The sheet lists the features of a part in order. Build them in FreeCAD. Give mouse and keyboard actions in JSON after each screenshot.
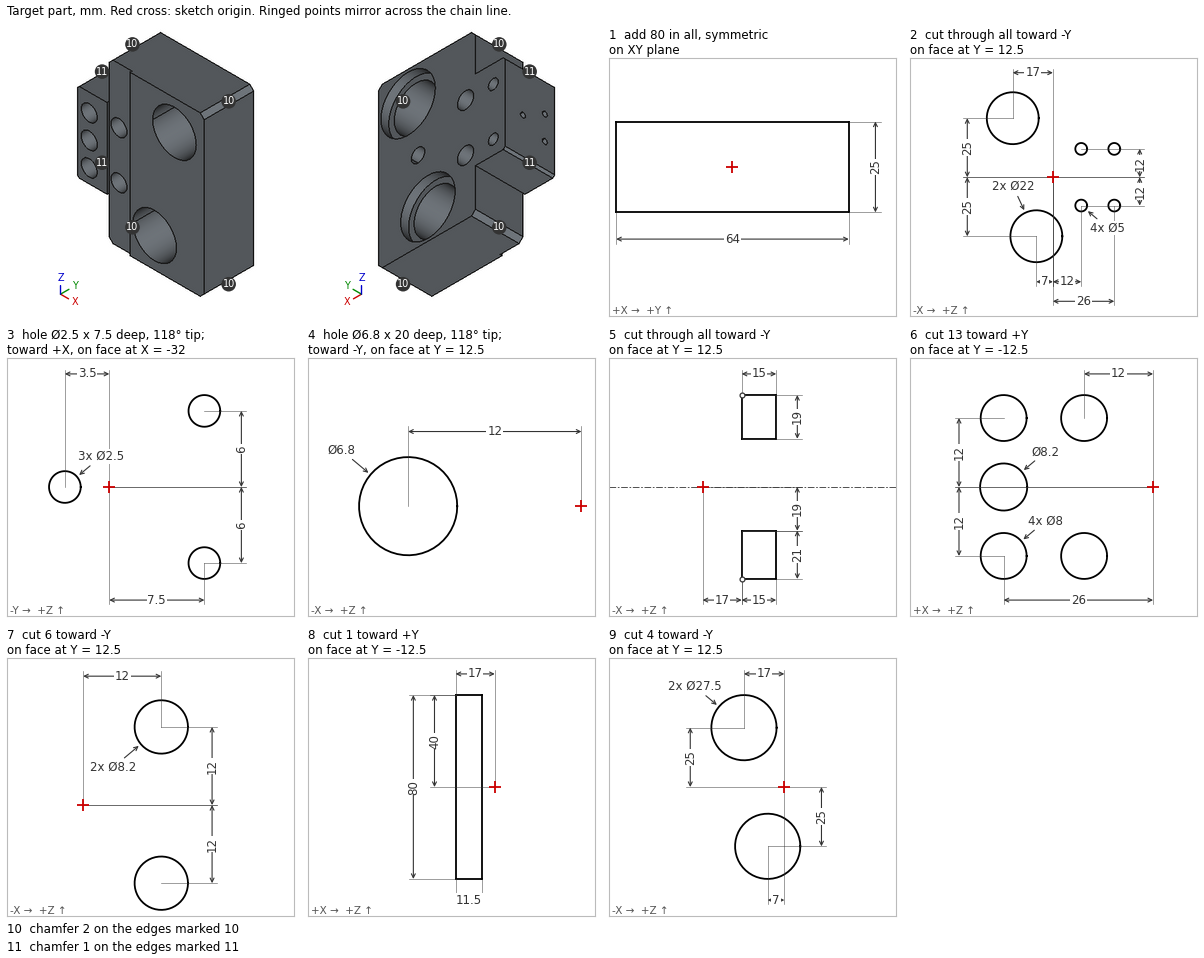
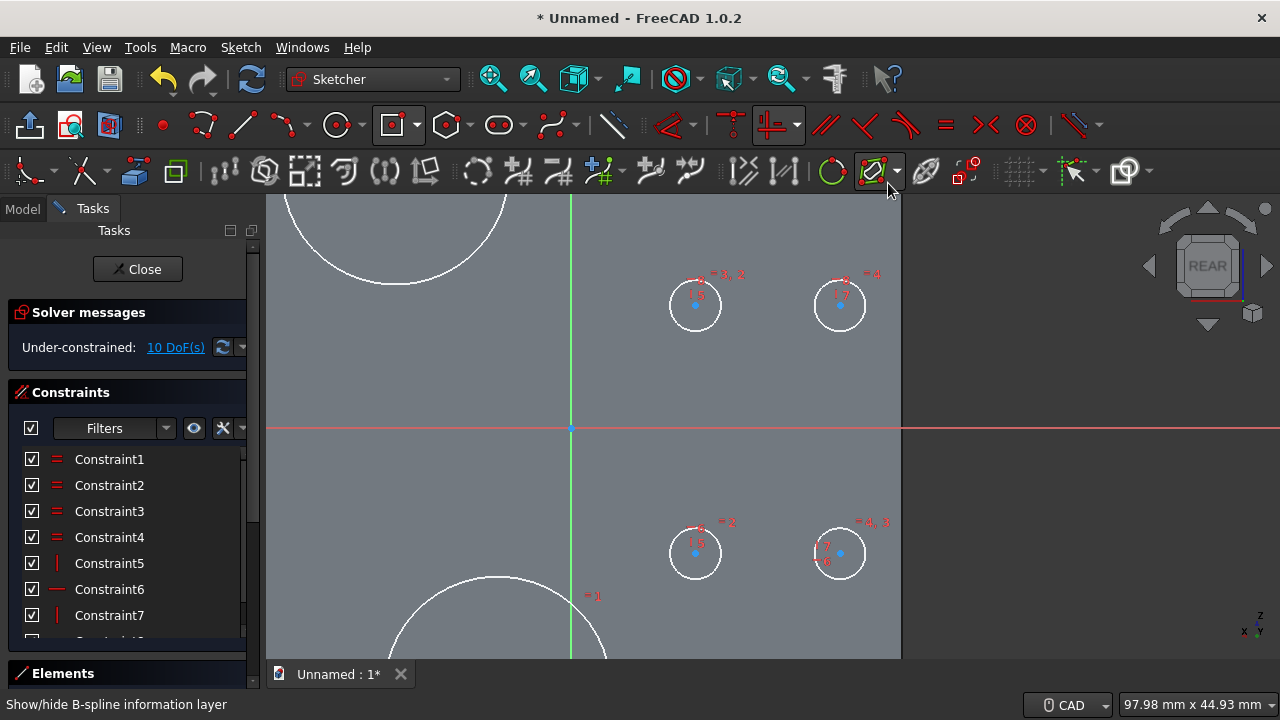
{"action": "left_click", "coordinate": [668, 126]}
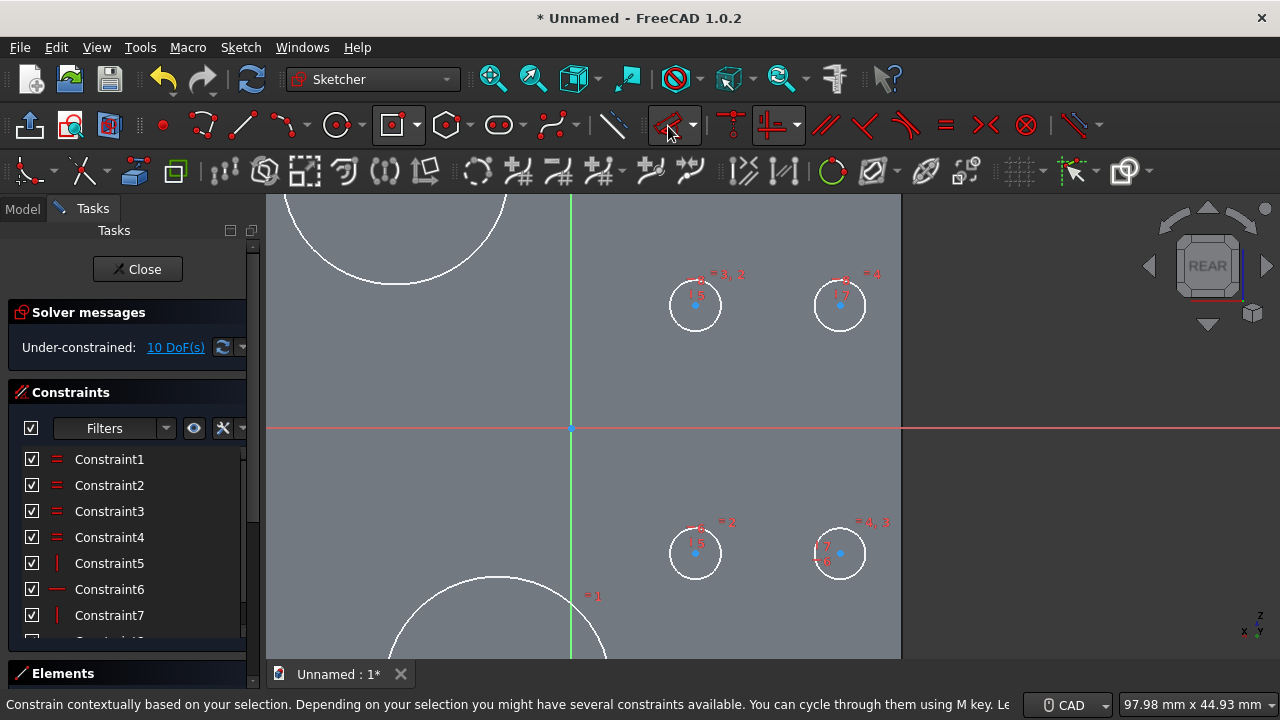
{"action": "left_click", "coordinate": [417, 610]}
{"action": "left_click", "coordinate": [394, 587]}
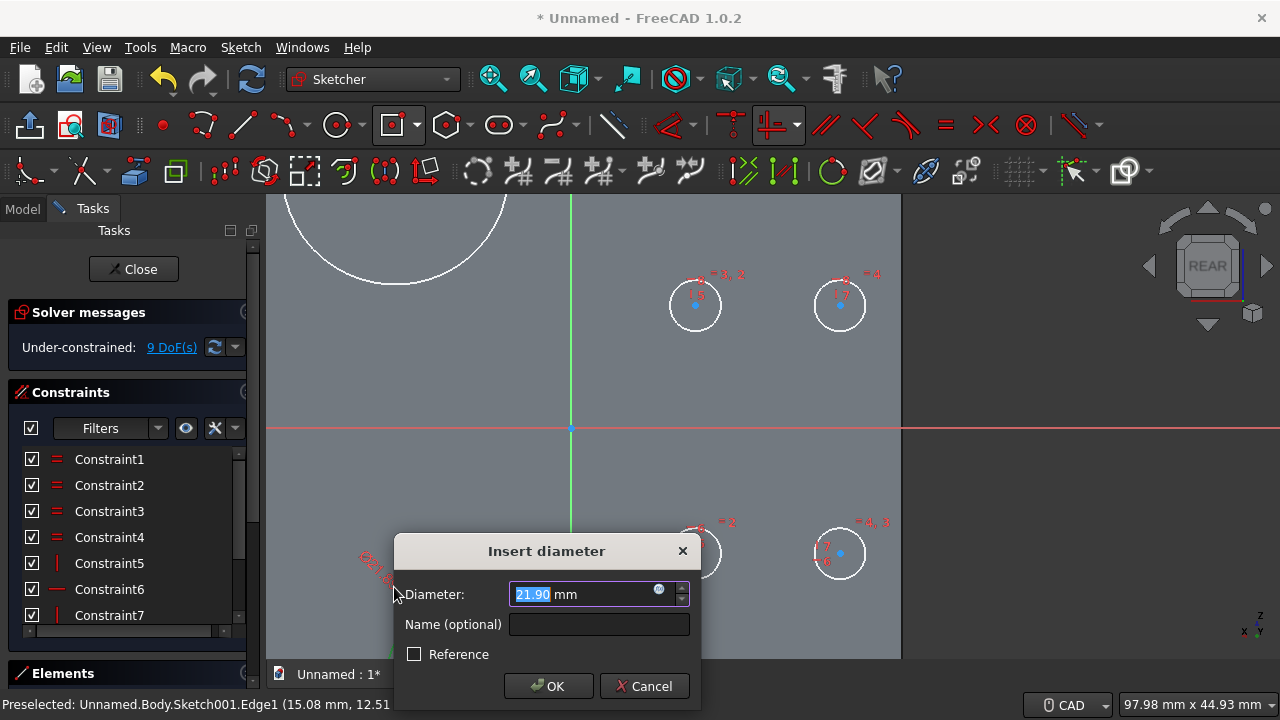
{"action": "type", "text": "22"}
{"action": "key", "text": "Return"}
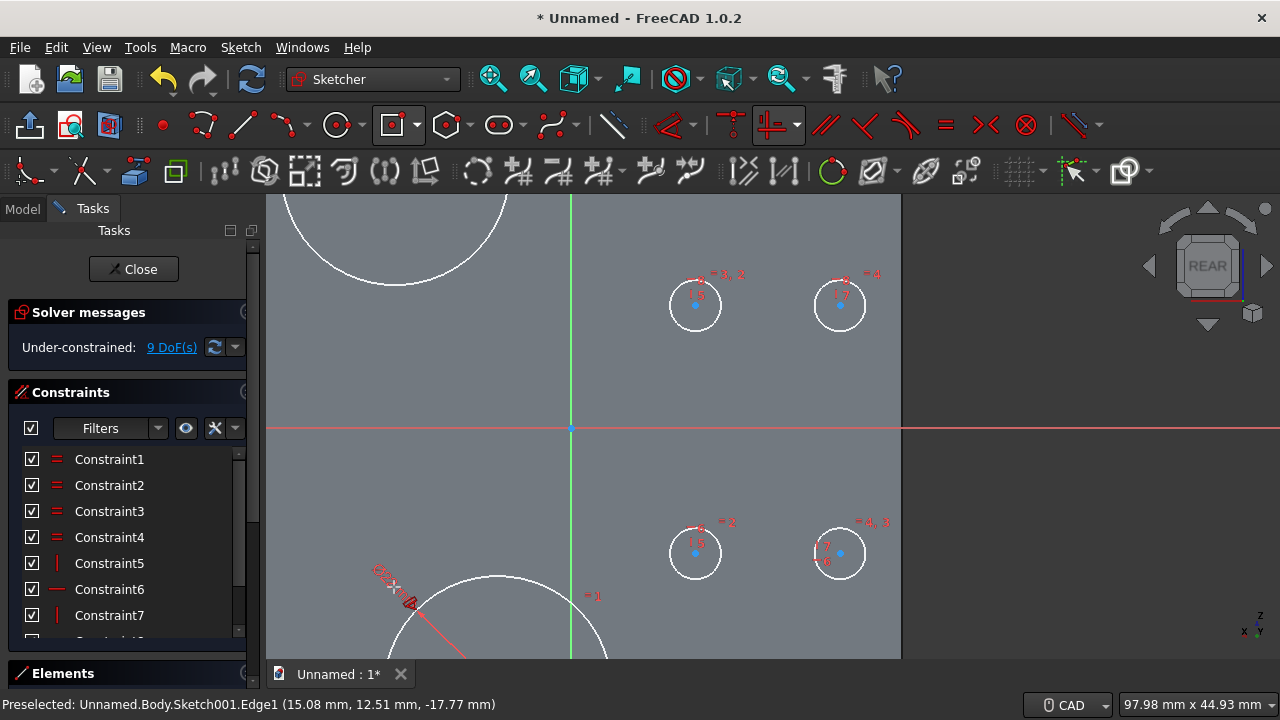
{"action": "left_click", "coordinate": [713, 536]}
{"action": "left_click", "coordinate": [736, 513]}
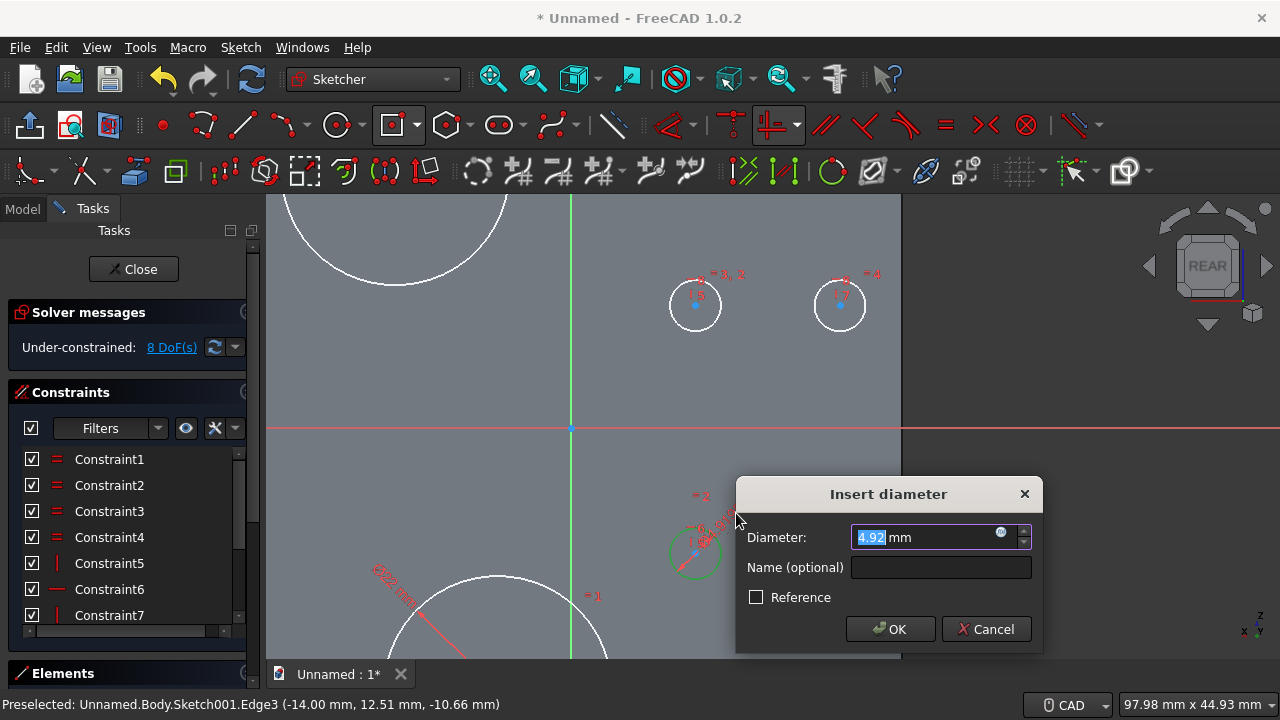
{"action": "type", "text": "5"}
{"action": "key", "text": "Return"}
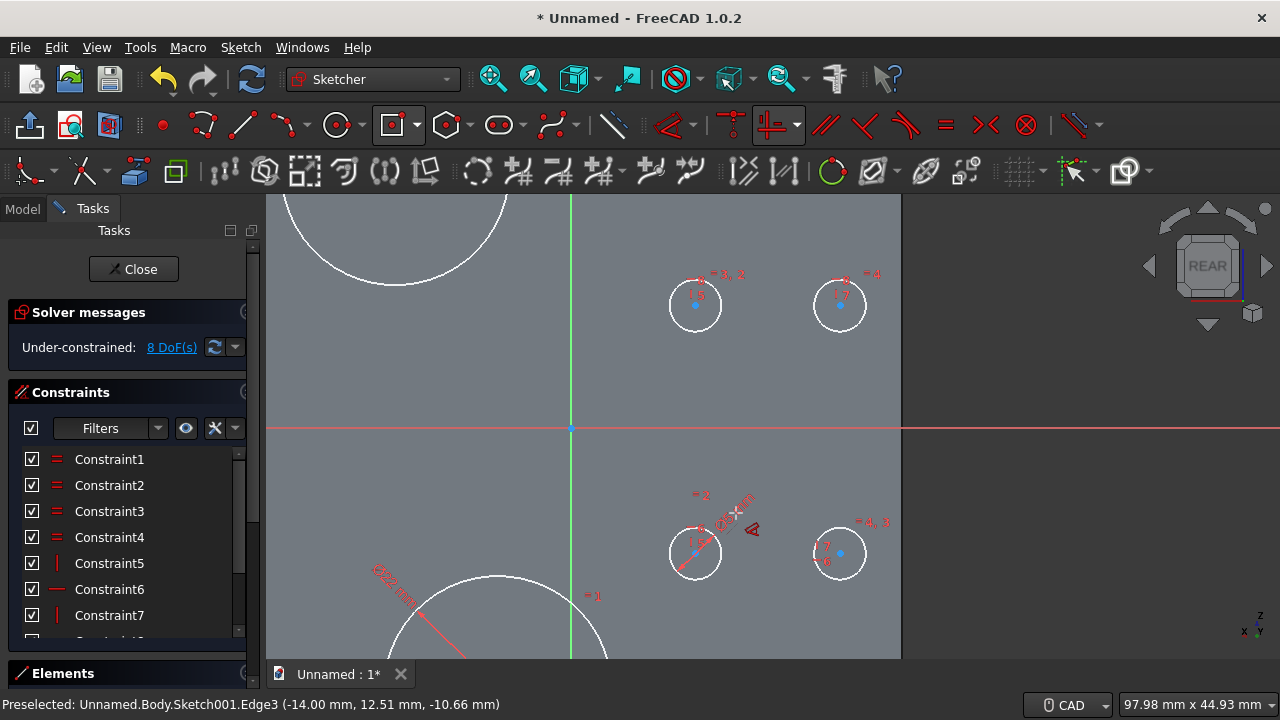
{"action": "scroll", "coordinate": [781, 425], "scroll_direction": "down", "scroll_amount": 5}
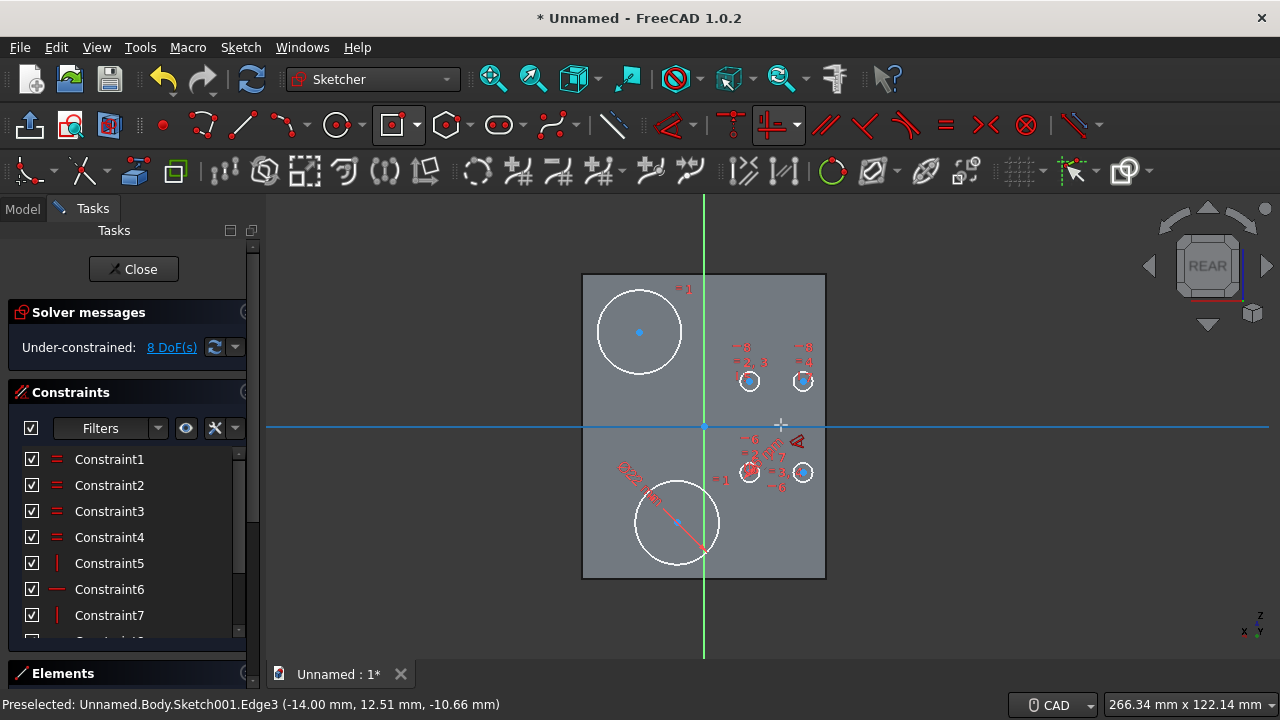
{"action": "scroll", "coordinate": [677, 523], "scroll_direction": "up", "scroll_amount": 2}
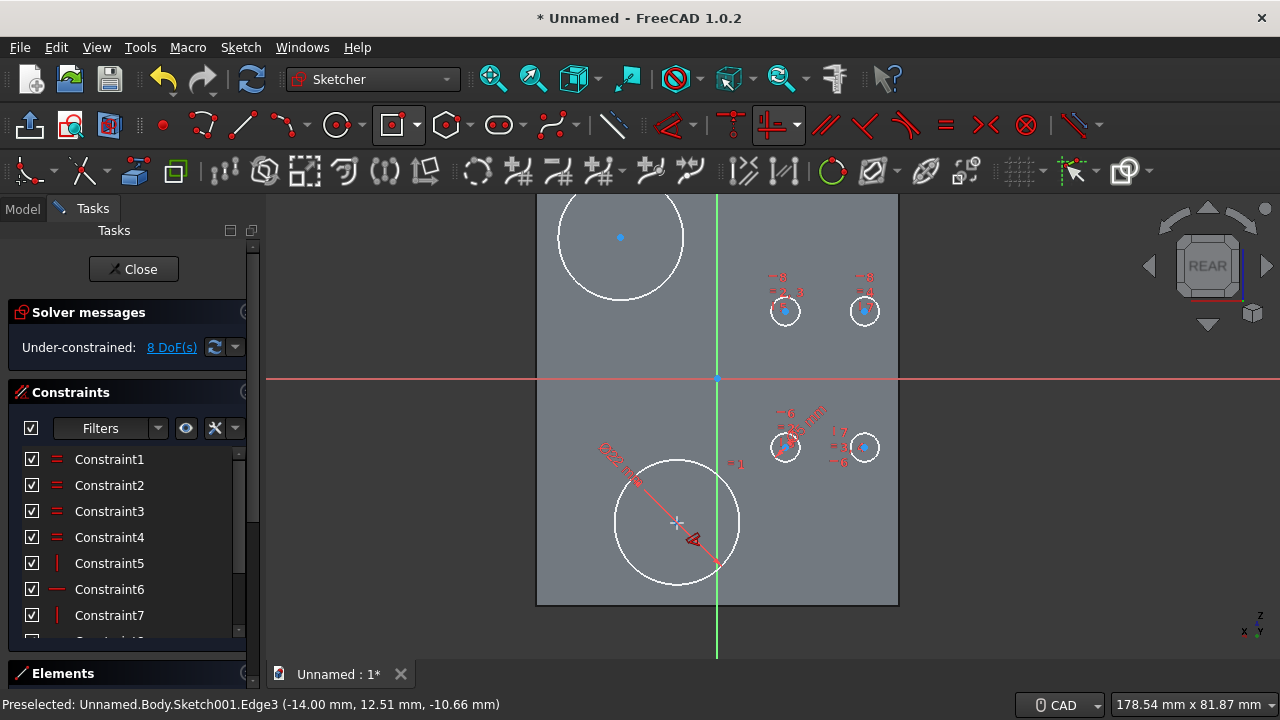
{"action": "left_click", "coordinate": [677, 522]}
{"action": "left_click", "coordinate": [697, 556]}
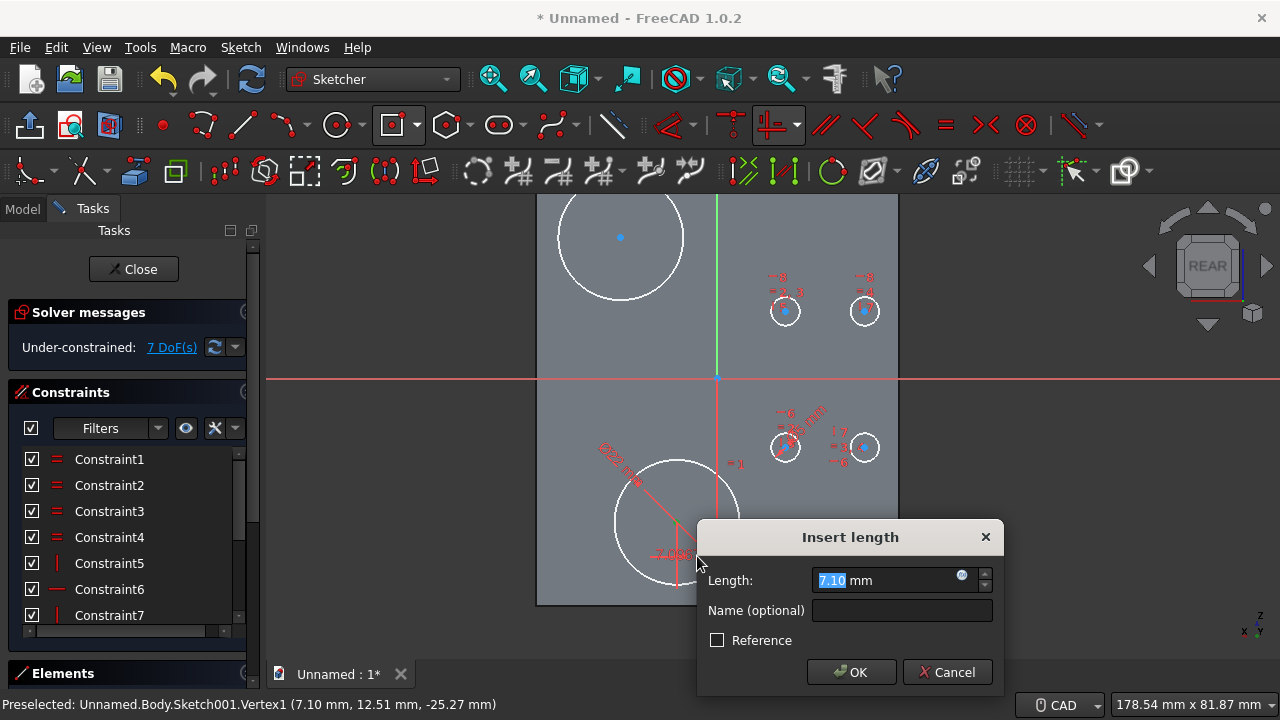
{"action": "type", "text": "7"}
{"action": "key", "text": "Return"}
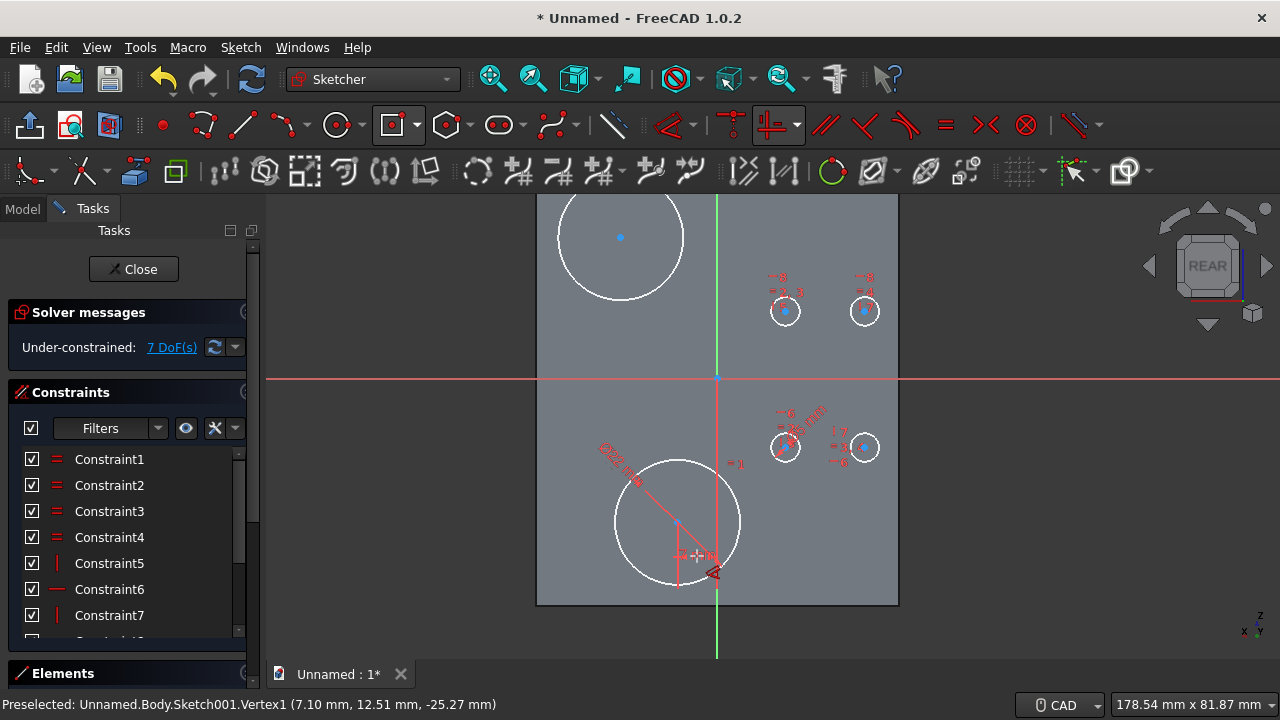
{"action": "left_click", "coordinate": [678, 522]}
{"action": "left_click", "coordinate": [644, 418]}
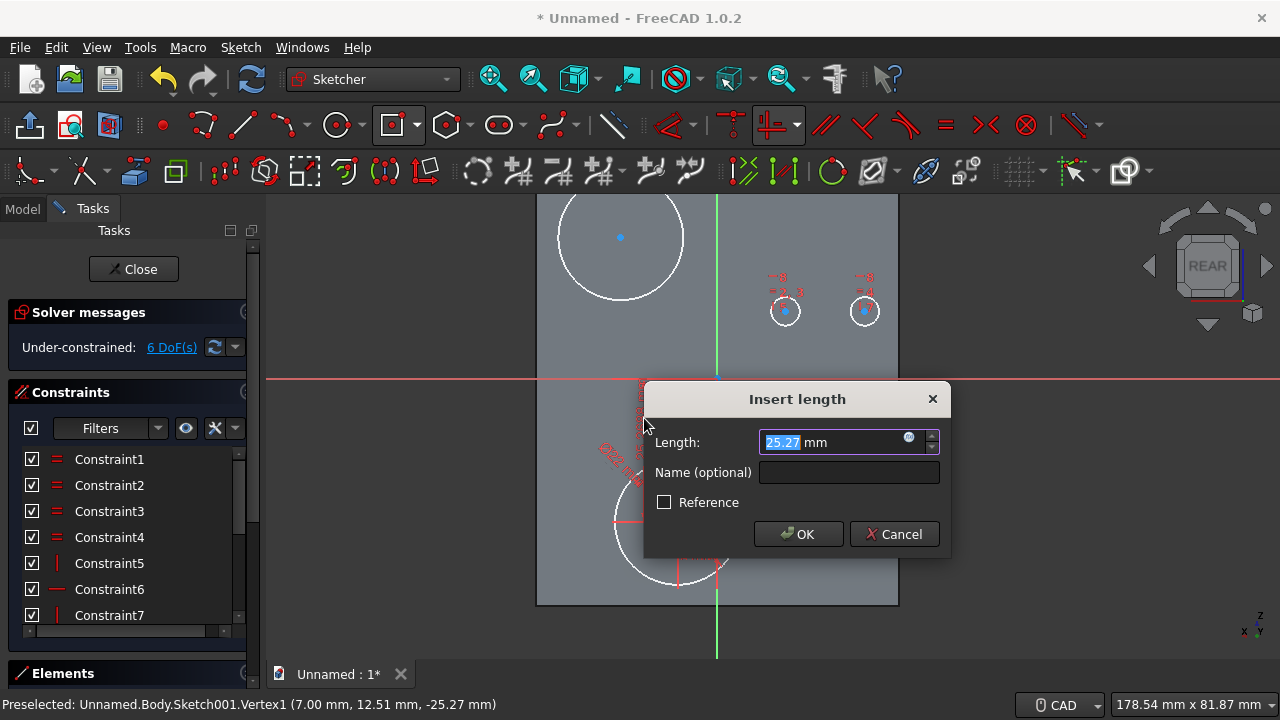
{"action": "type", "text": "25"}
{"action": "key", "text": "Return"}